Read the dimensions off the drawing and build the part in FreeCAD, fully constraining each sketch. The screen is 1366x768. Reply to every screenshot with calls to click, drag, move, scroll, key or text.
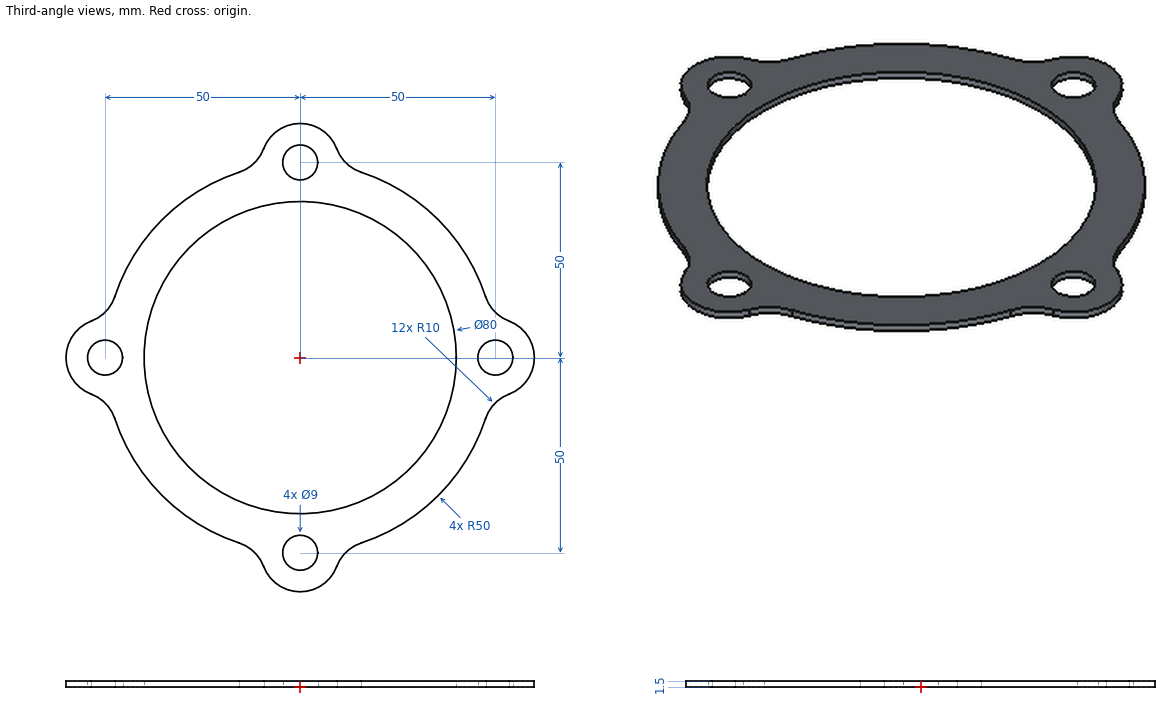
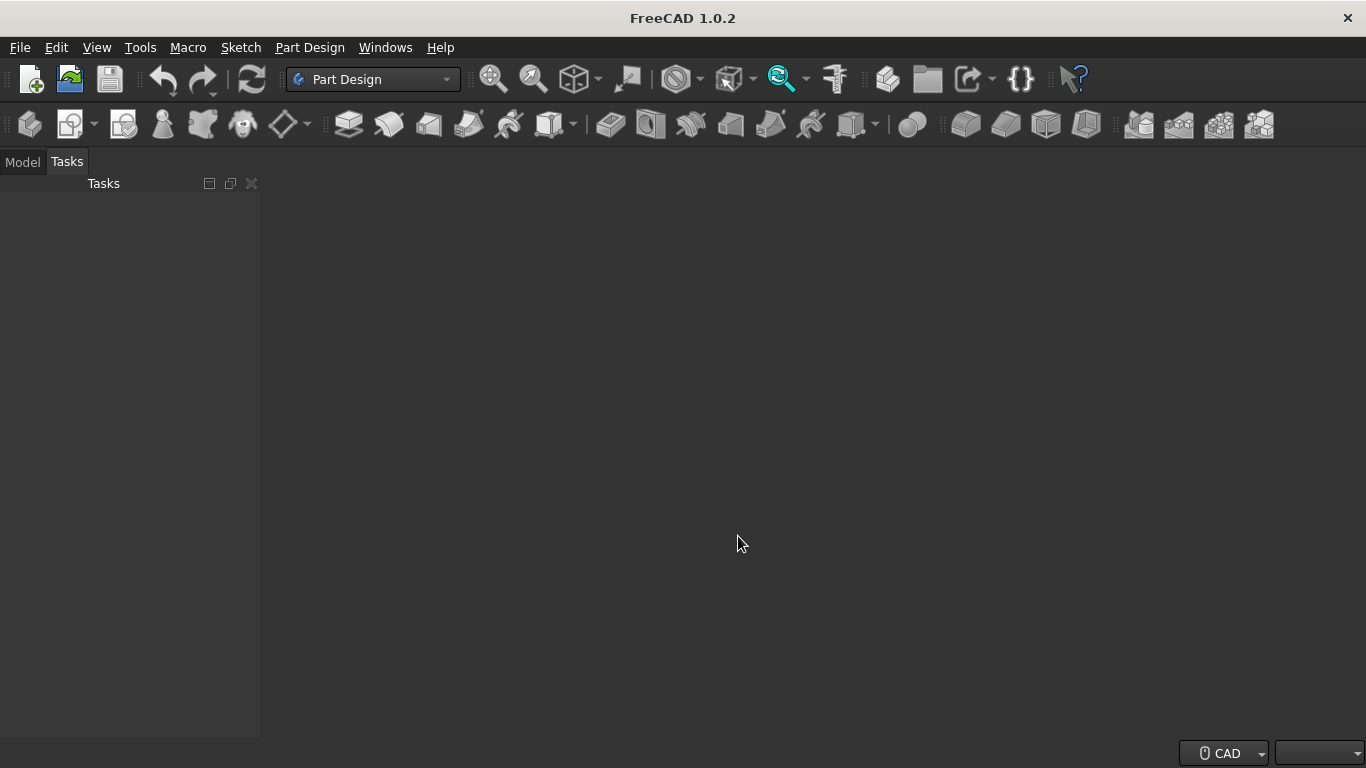
click(30, 80)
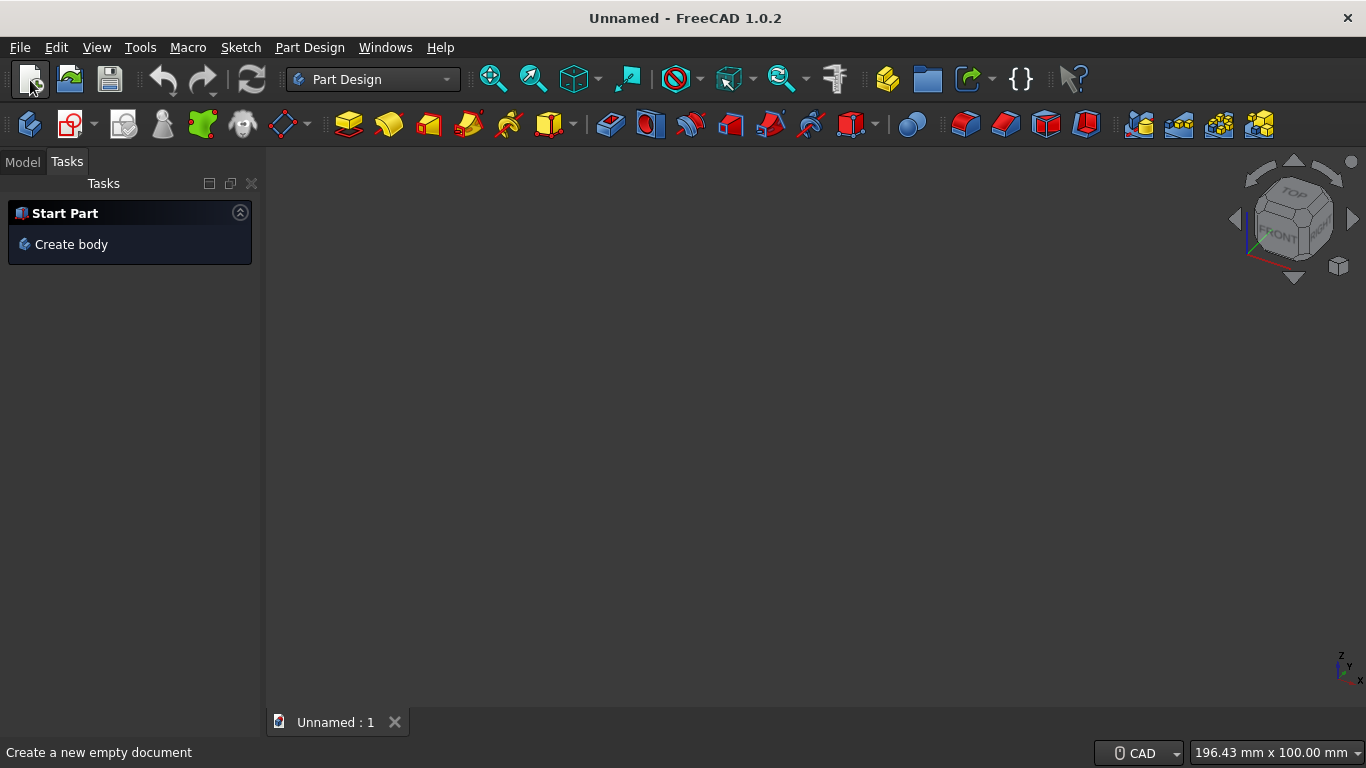
click(70, 124)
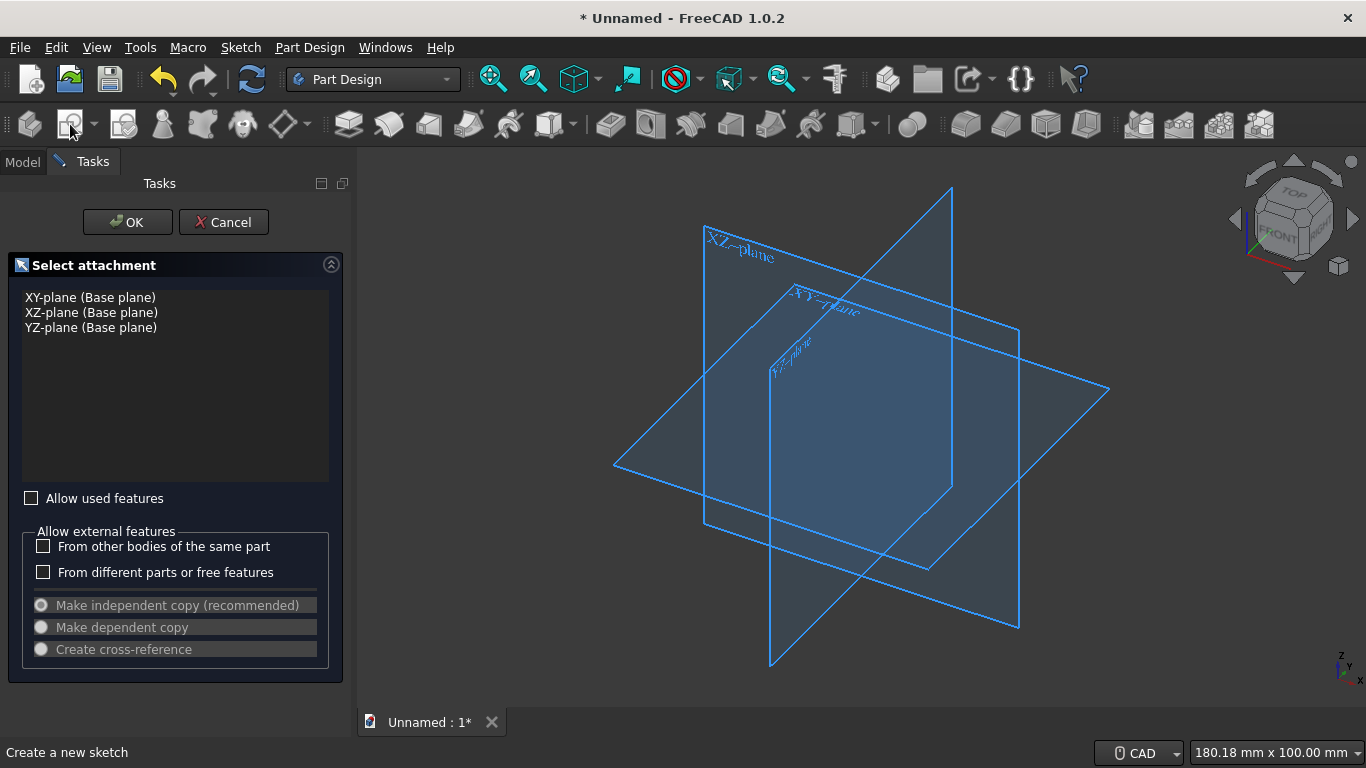
click(82, 298)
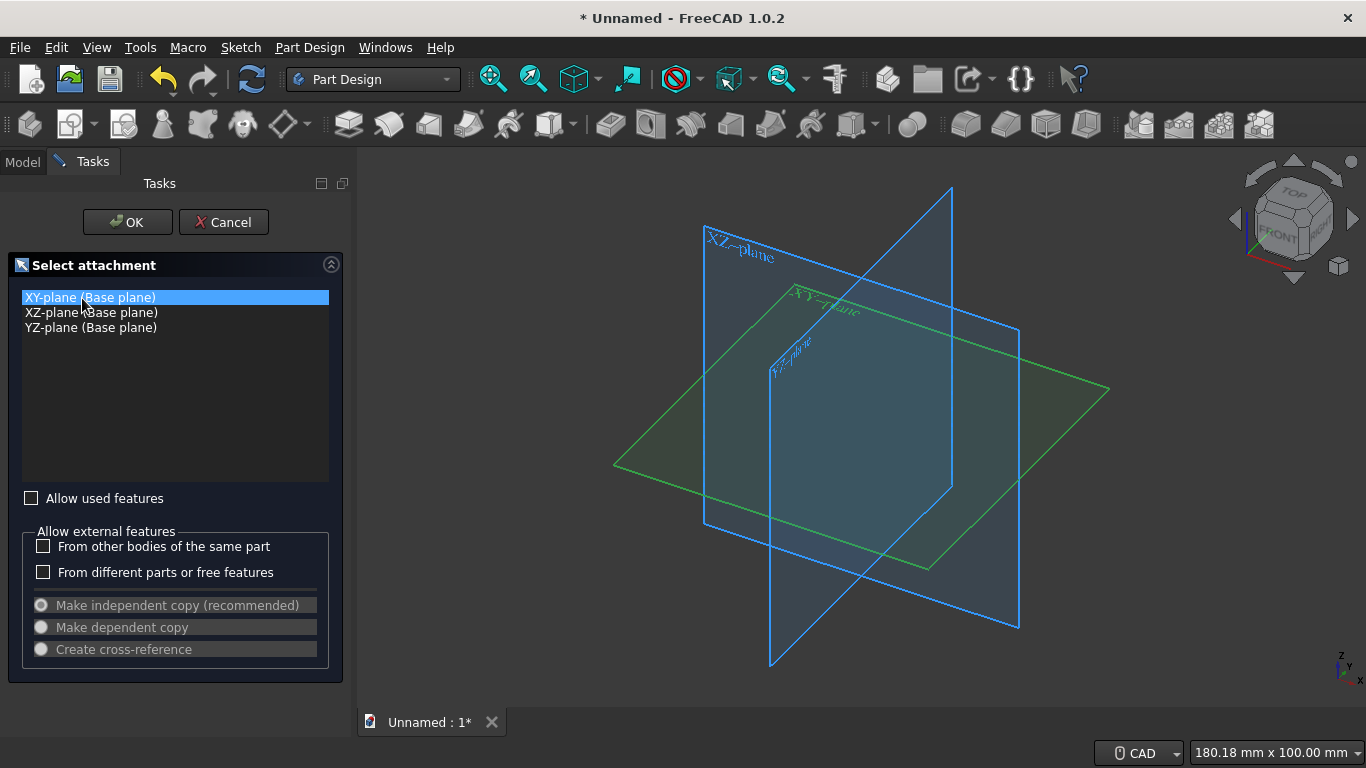
click(128, 222)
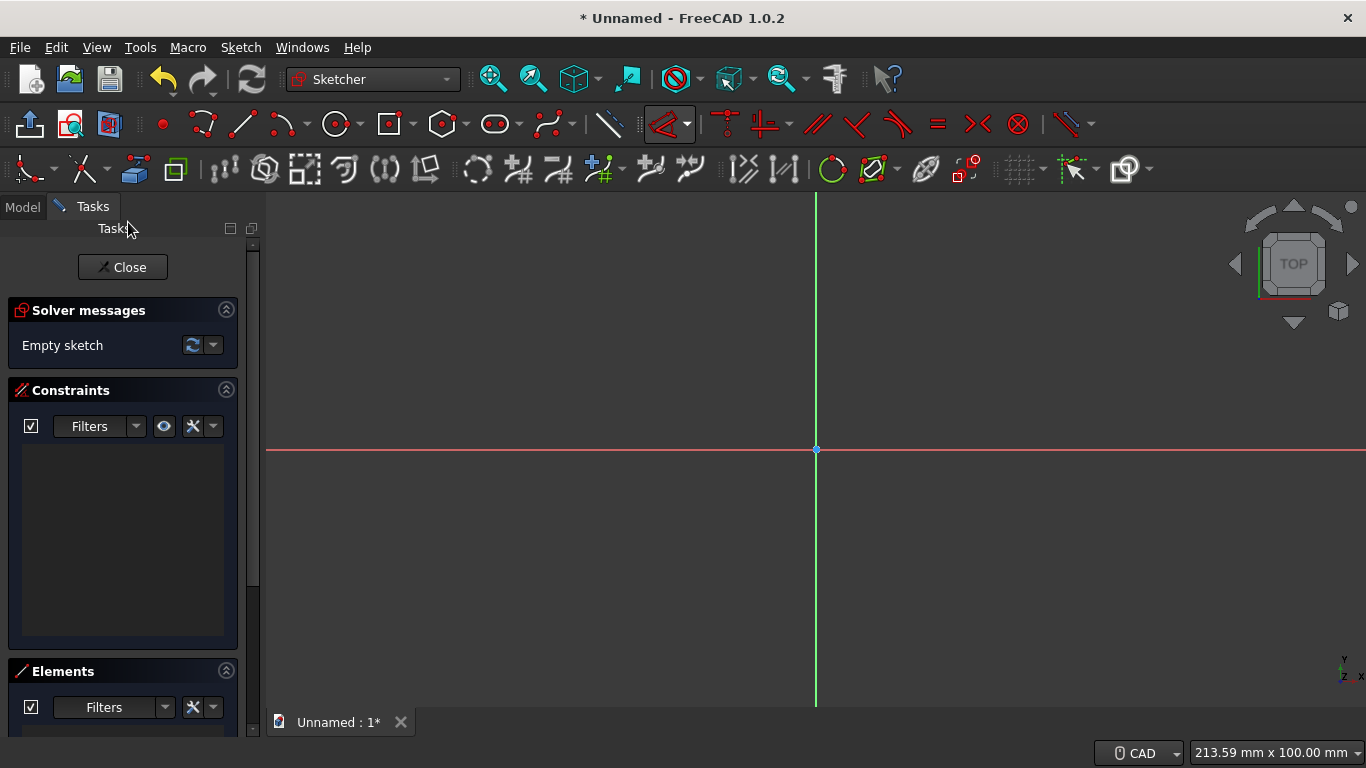
scroll(664, 450, down, 3)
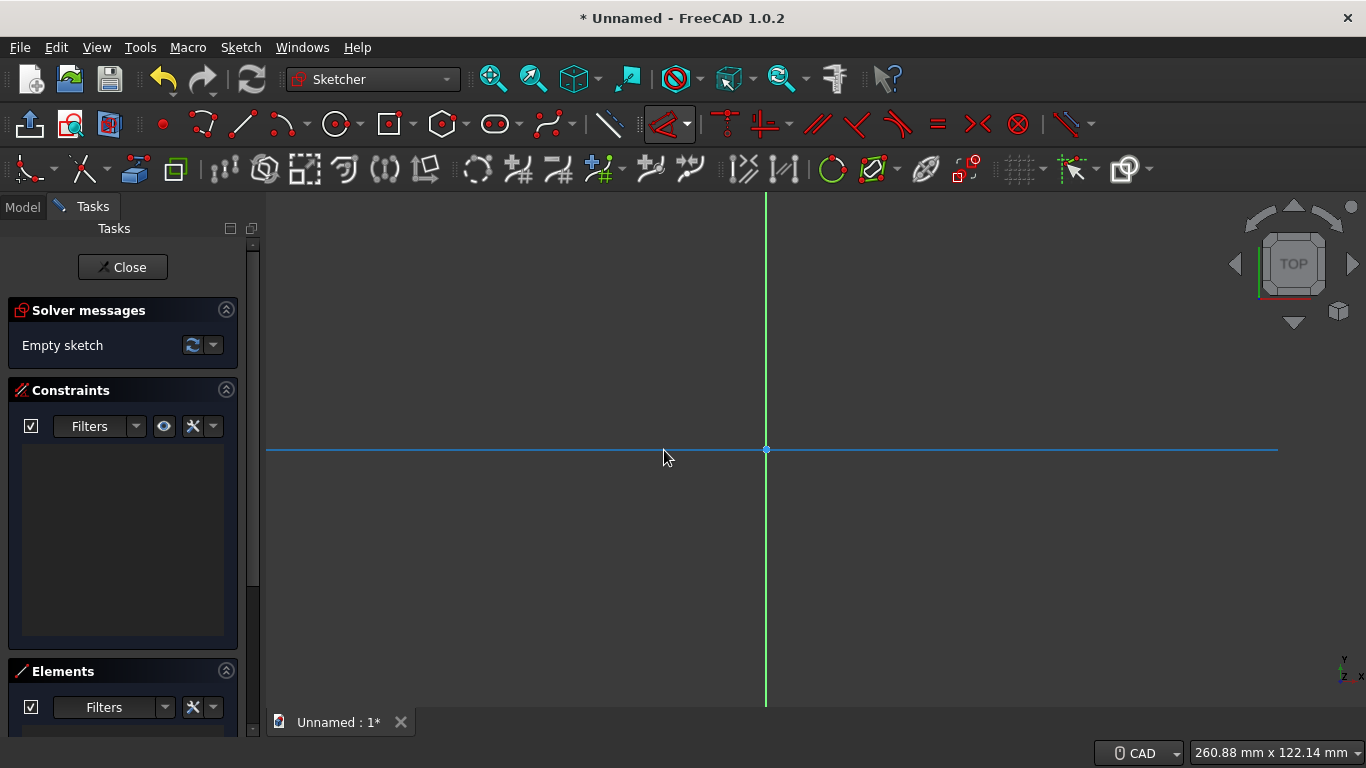
key(g)
key(3)
key(a)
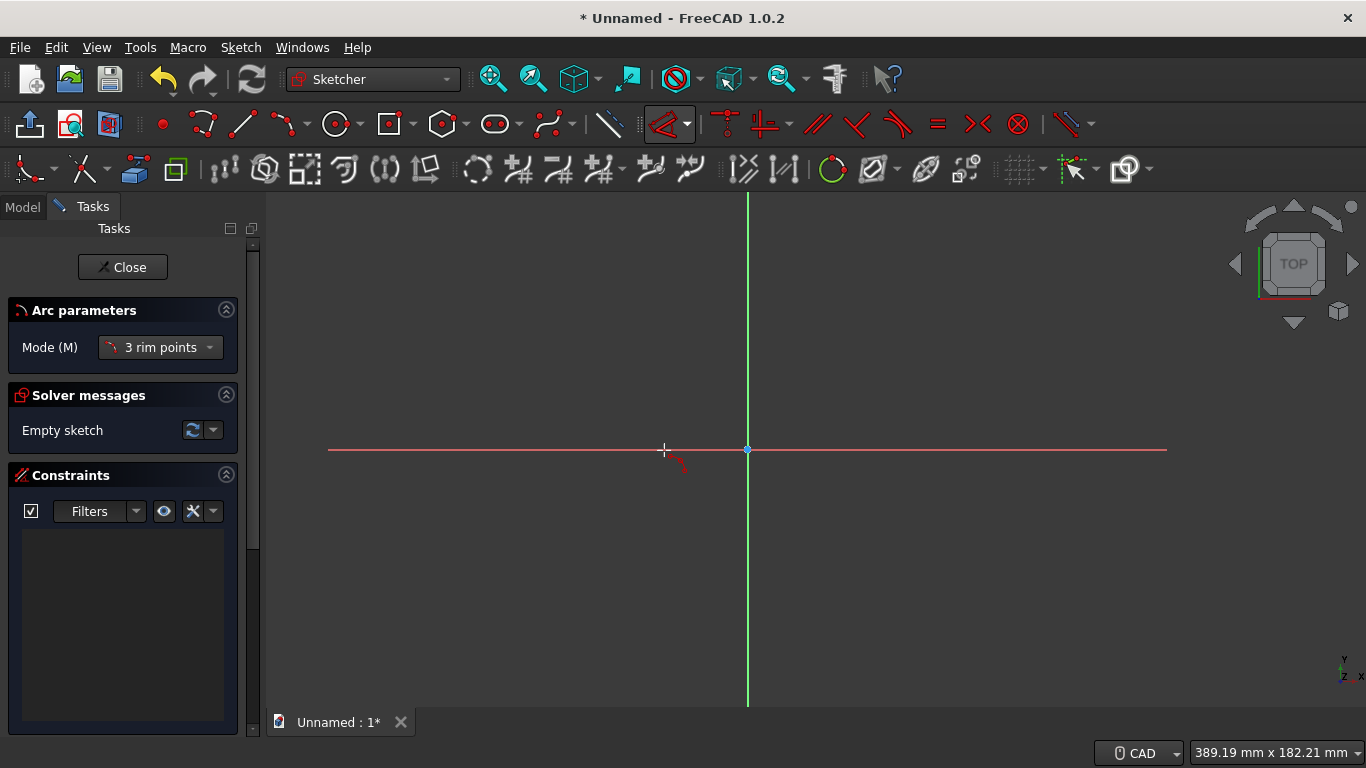
click(792, 584)
click(882, 494)
click(848, 550)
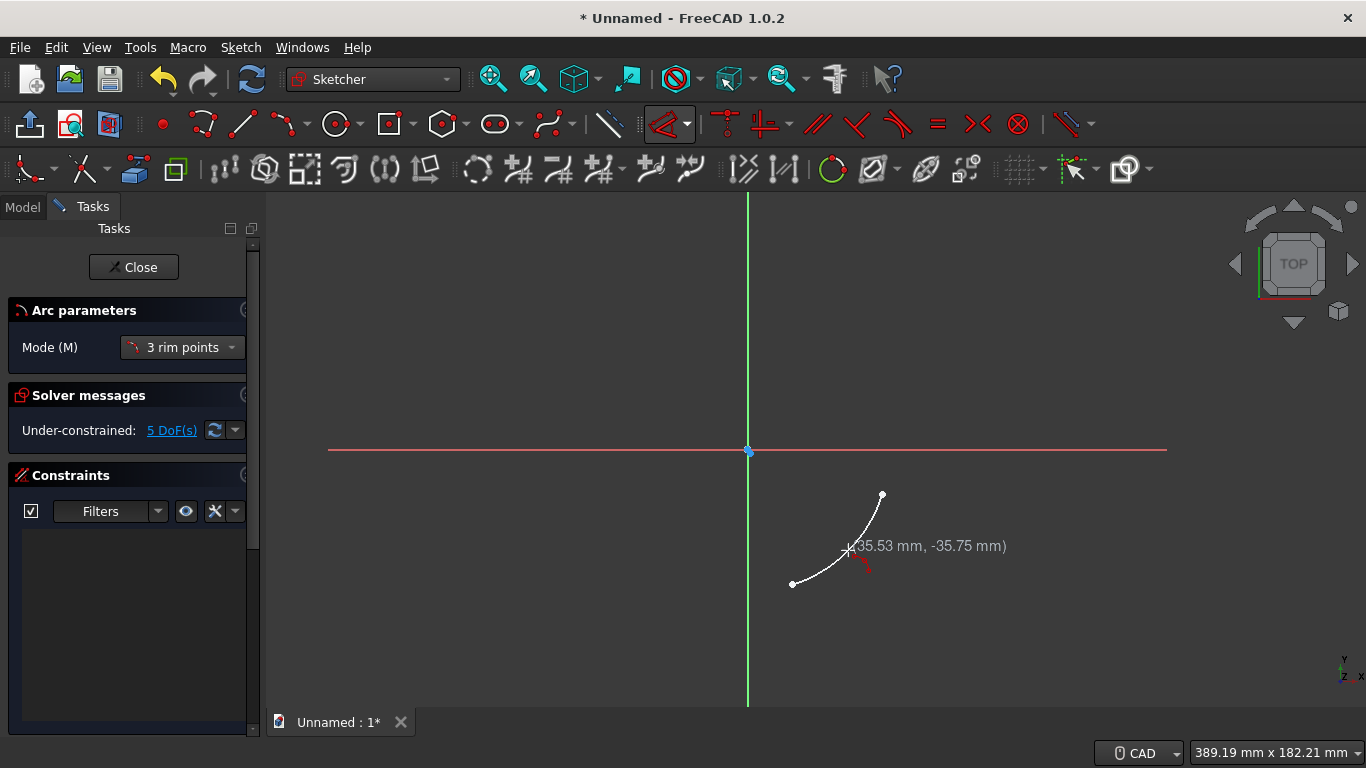
click(882, 495)
click(899, 476)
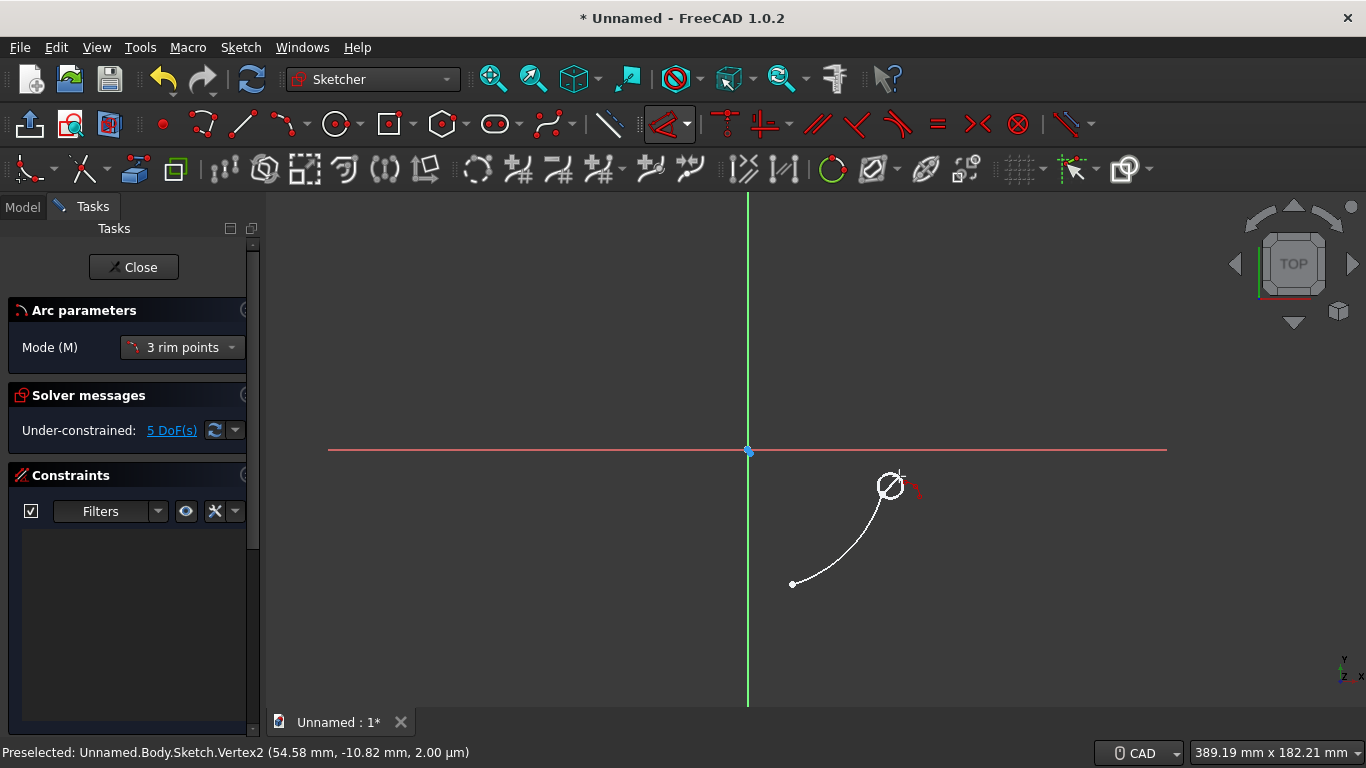
scroll(888, 483, up, 9)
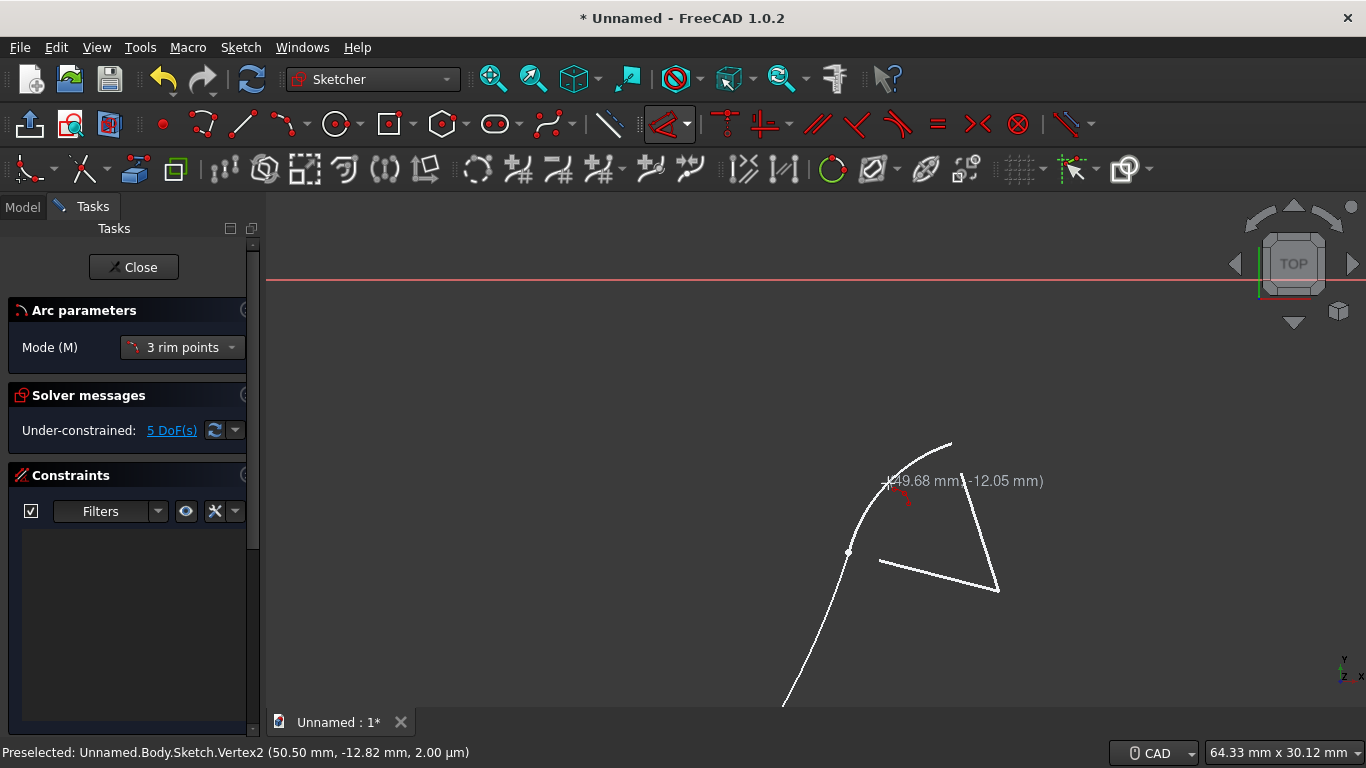
click(887, 482)